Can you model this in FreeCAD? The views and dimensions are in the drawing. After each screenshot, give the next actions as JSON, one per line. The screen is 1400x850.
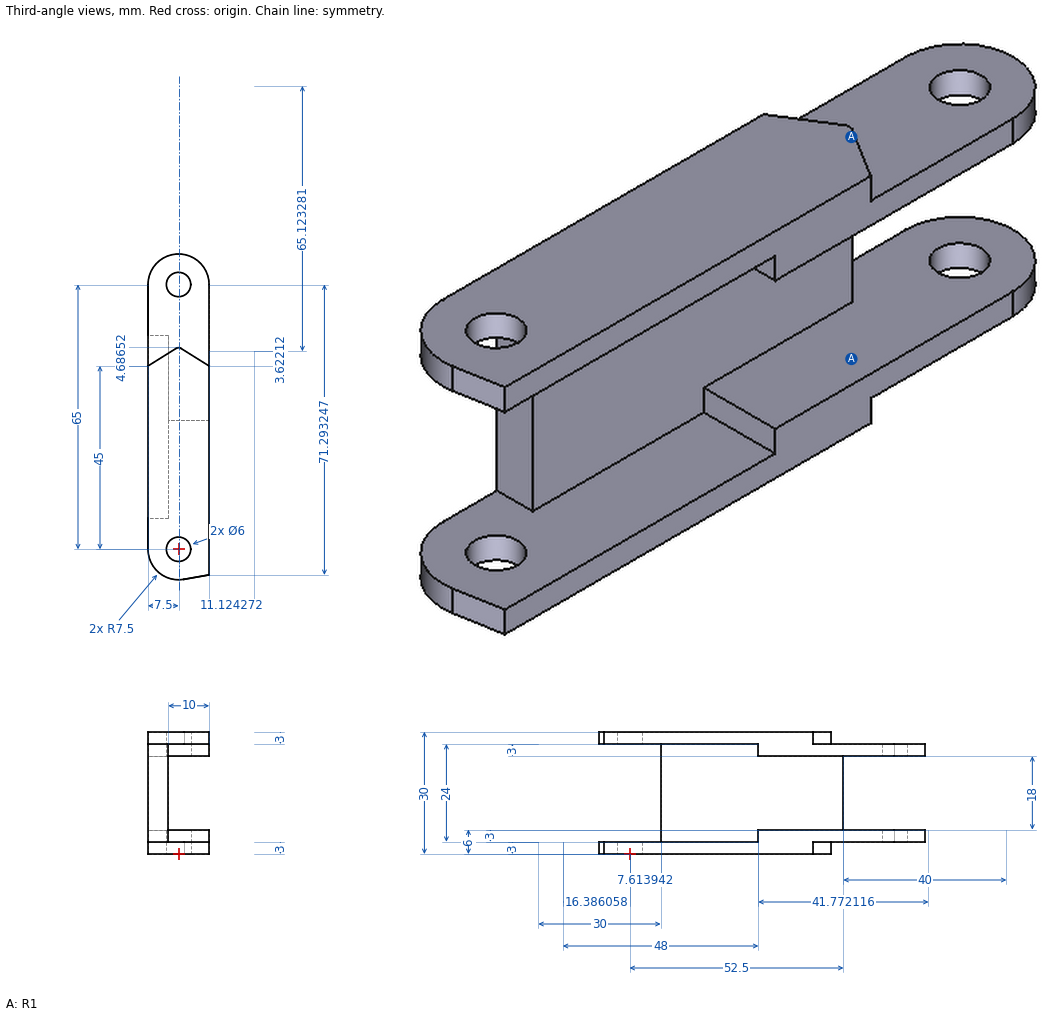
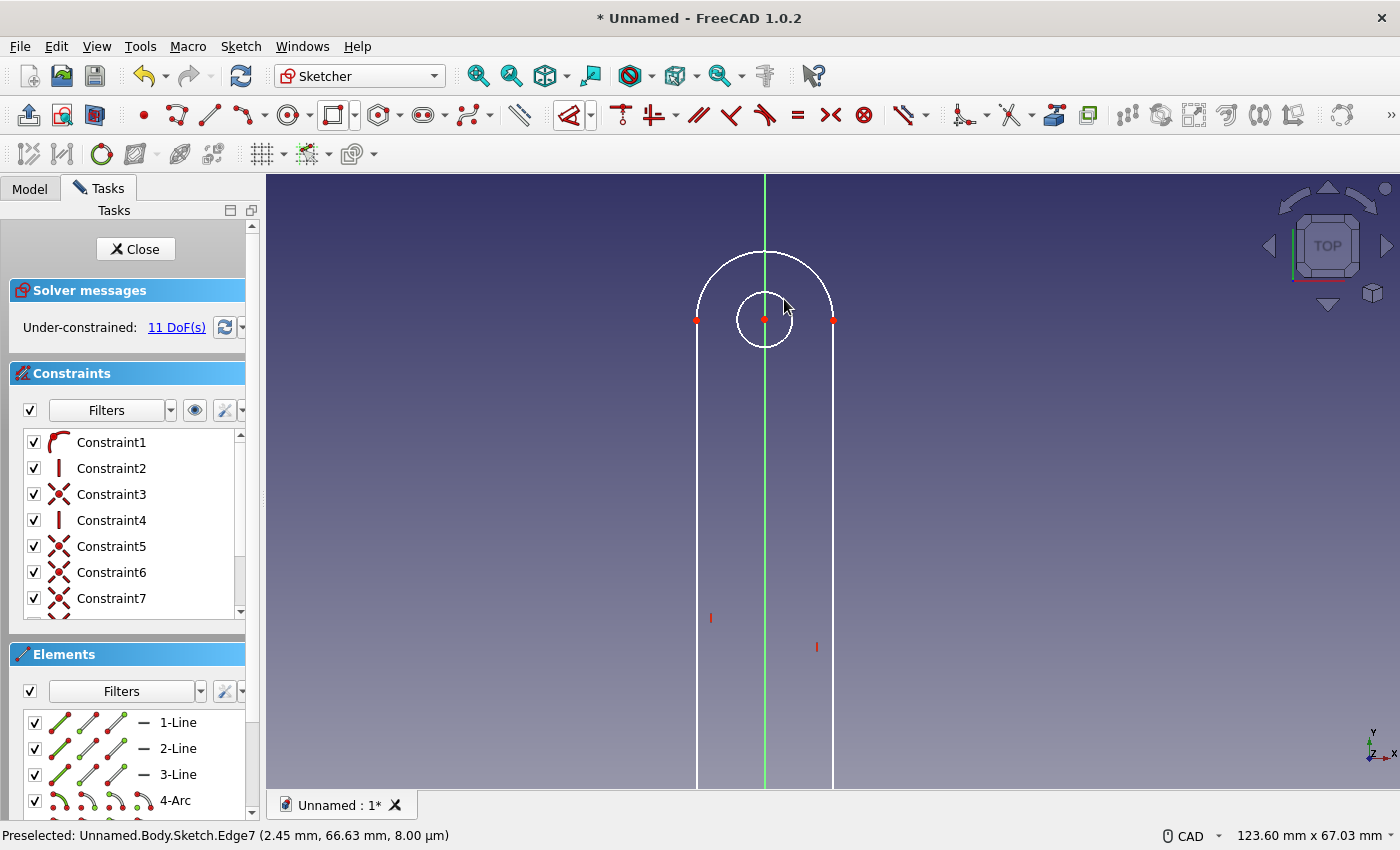
{"action": "left_click", "coordinate": [697, 499]}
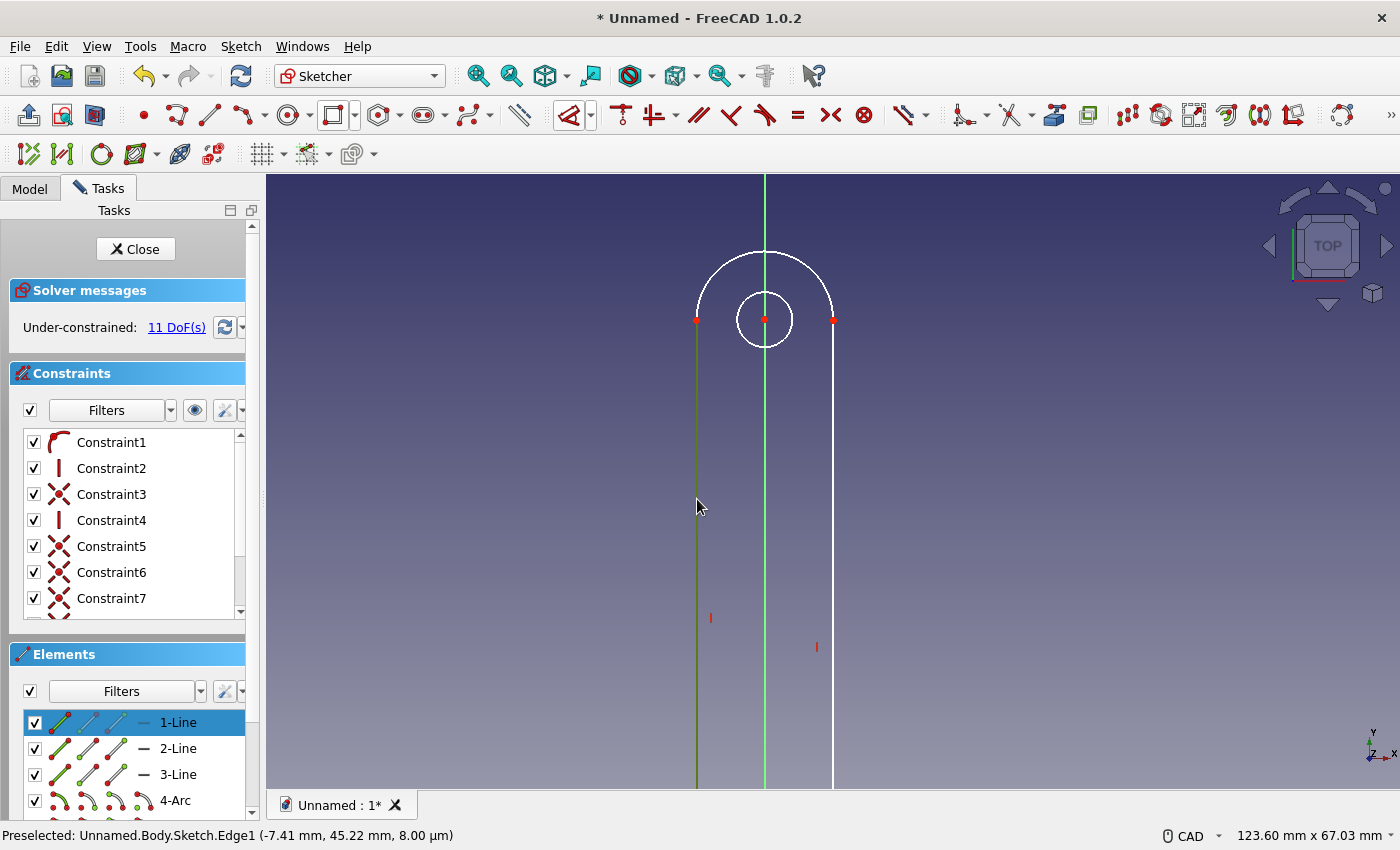
{"action": "scroll", "coordinate": [764, 318], "scroll_direction": "down", "scroll_amount": 3}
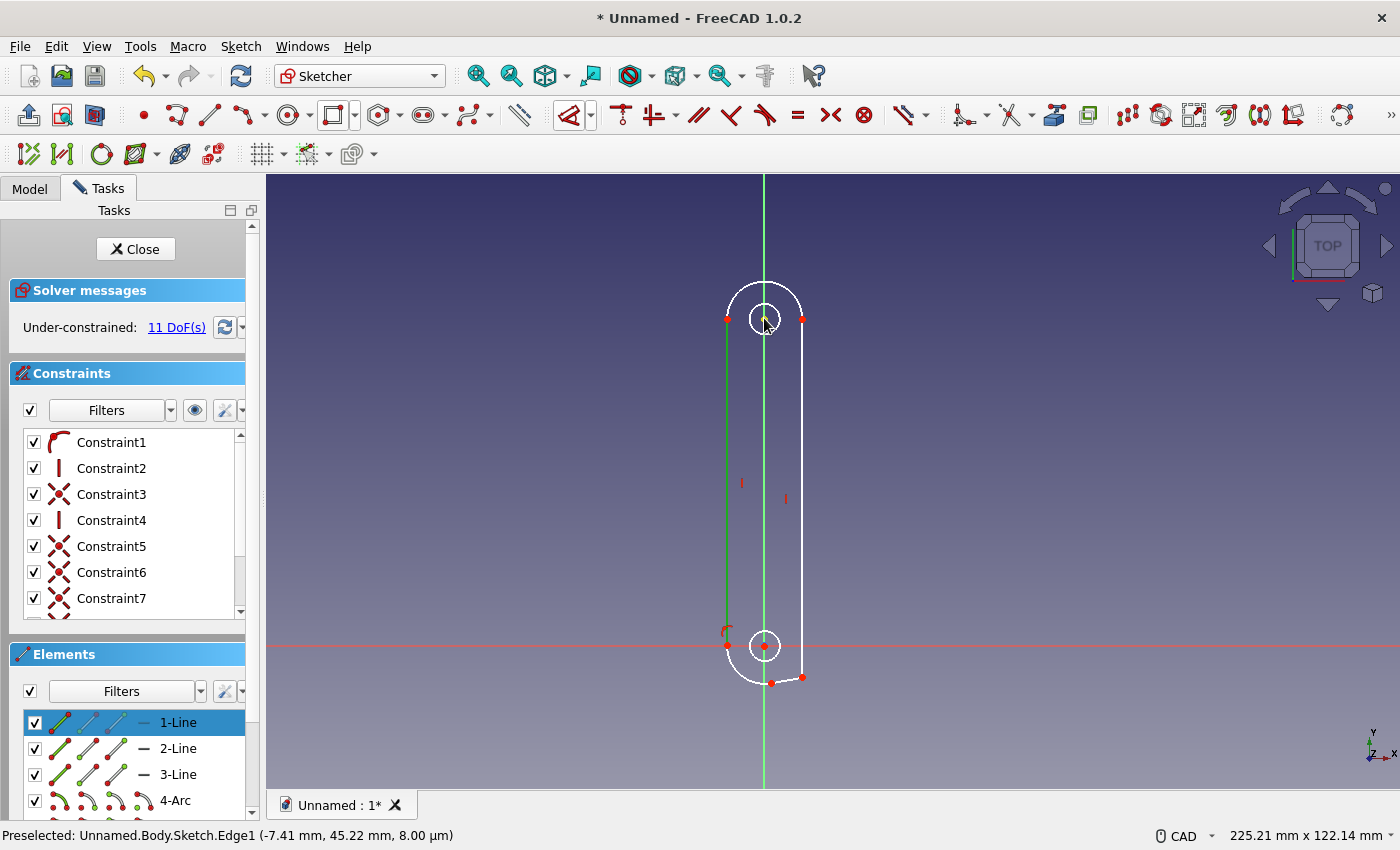
{"action": "left_click", "coordinate": [732, 665]}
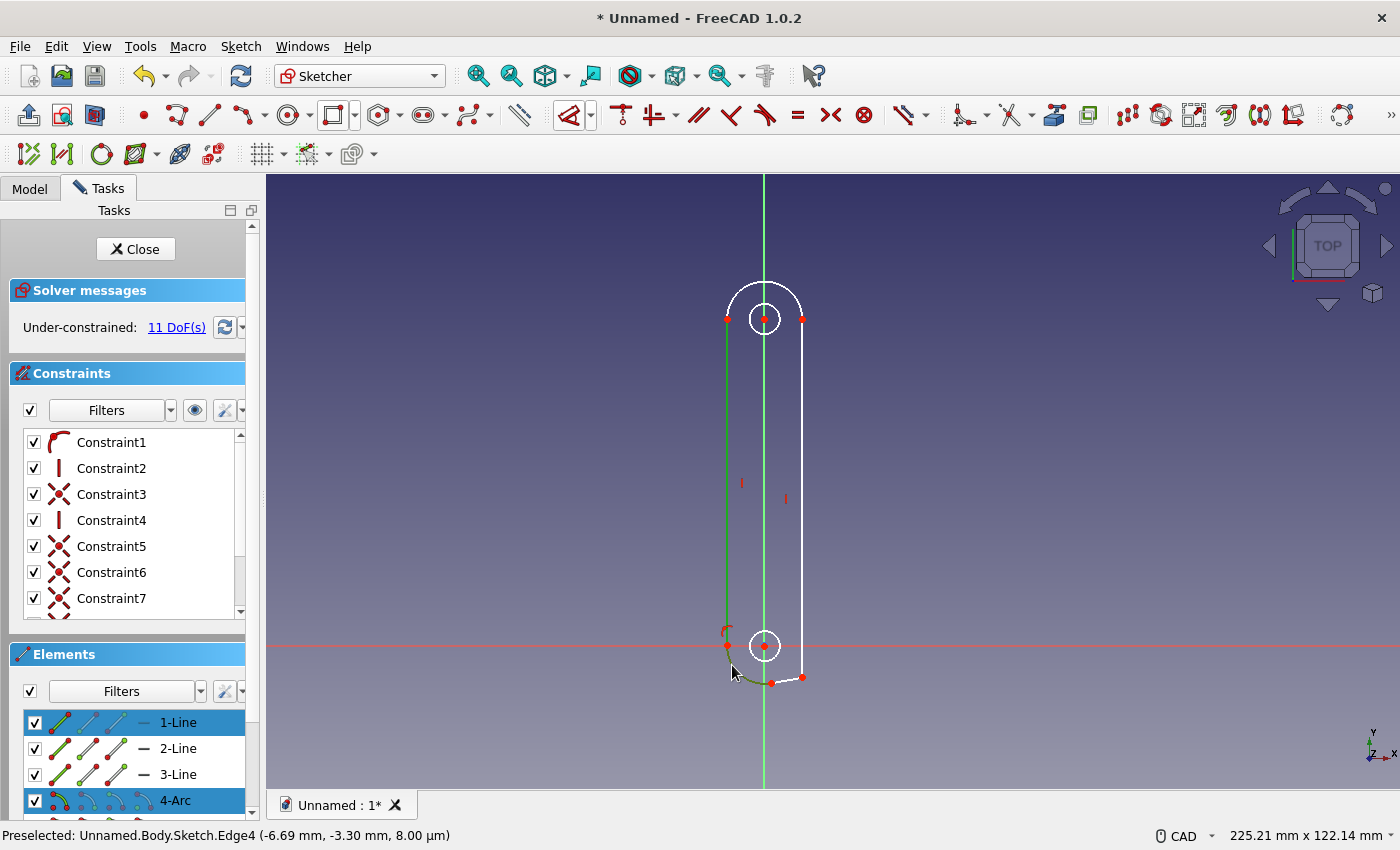
{"action": "key", "text": "t"}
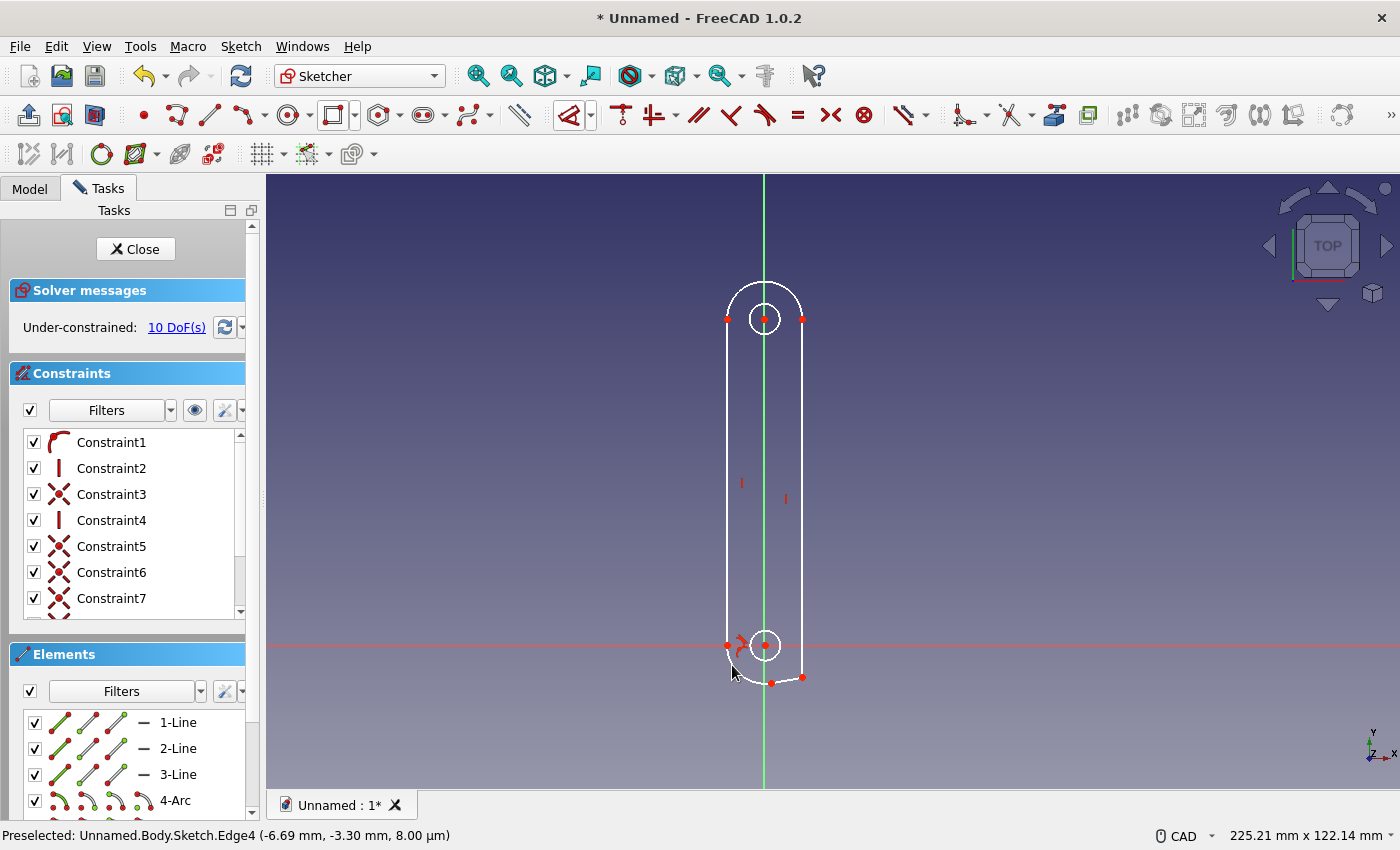
{"action": "left_click", "coordinate": [727, 417]}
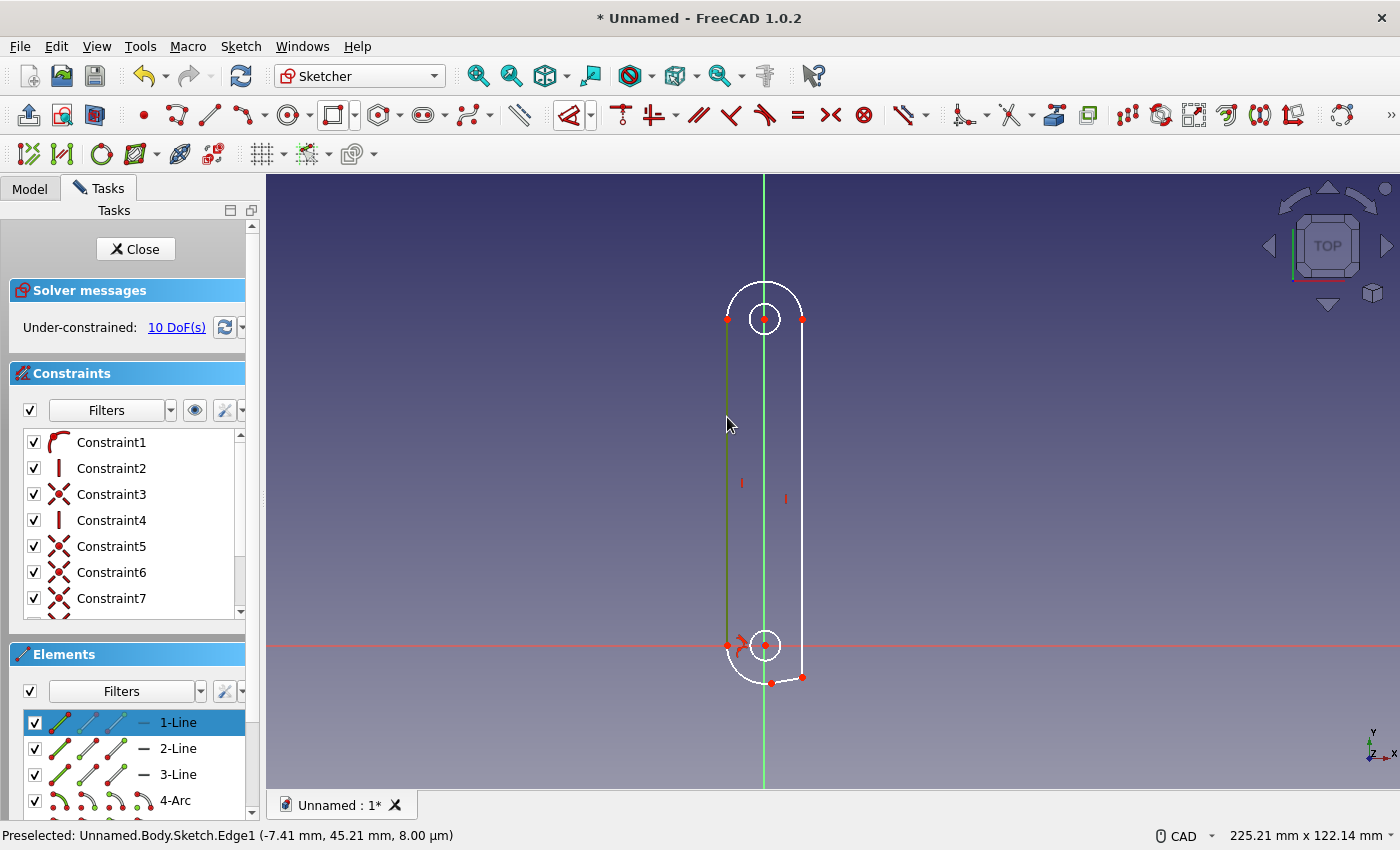
{"action": "left_click", "coordinate": [787, 289]}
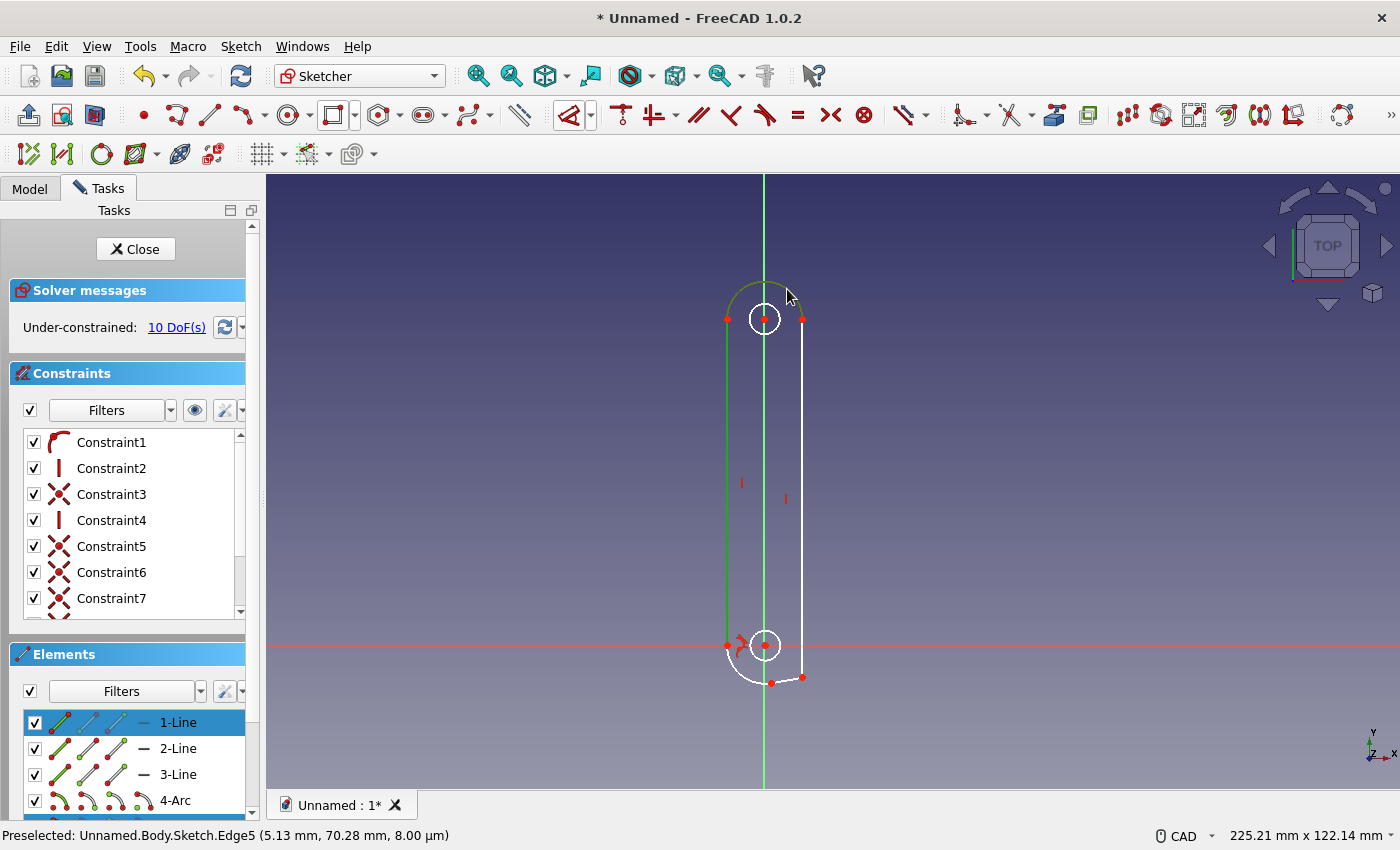
{"action": "key", "text": "t"}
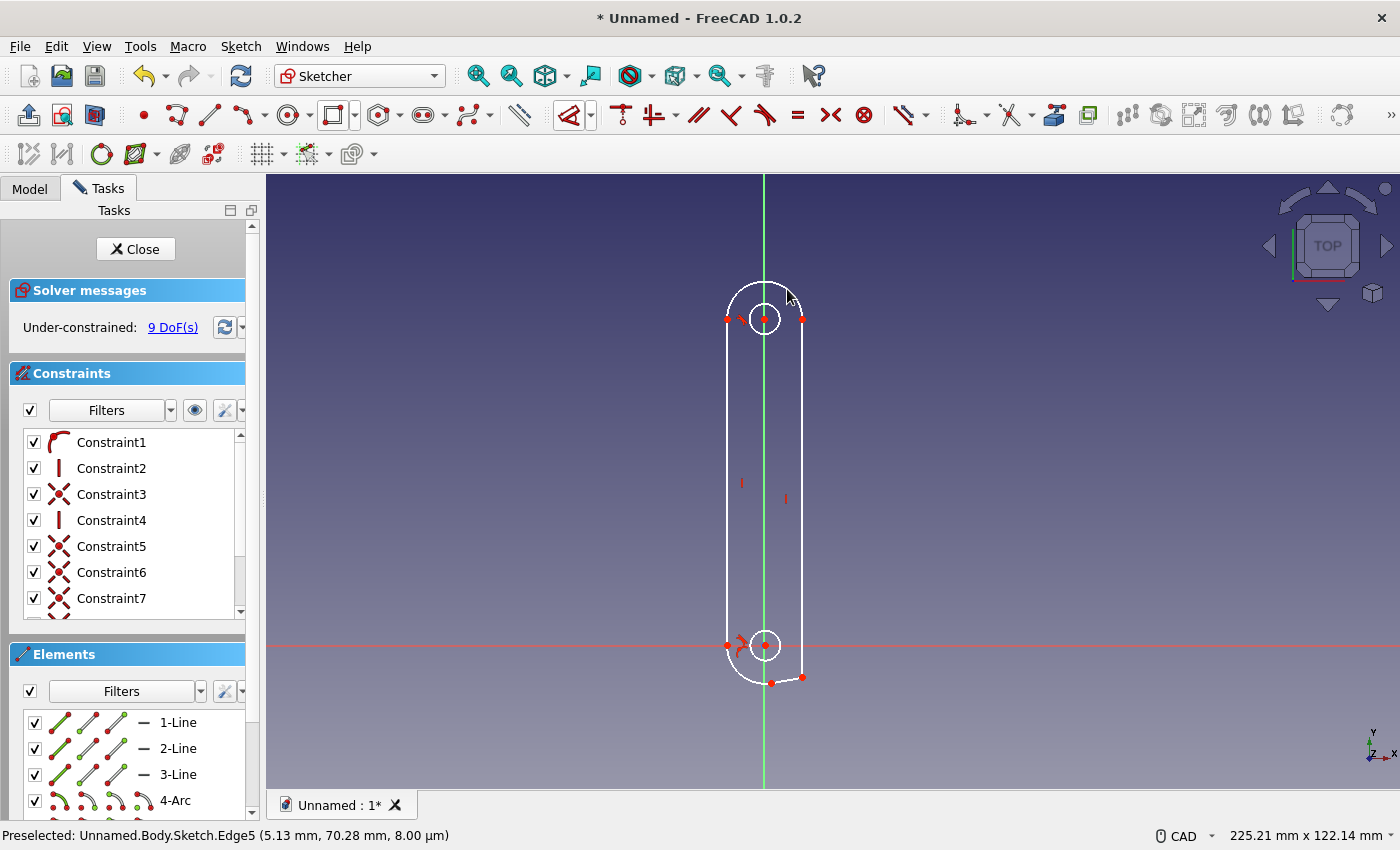
{"action": "scroll", "coordinate": [780, 682], "scroll_direction": "up", "scroll_amount": 2}